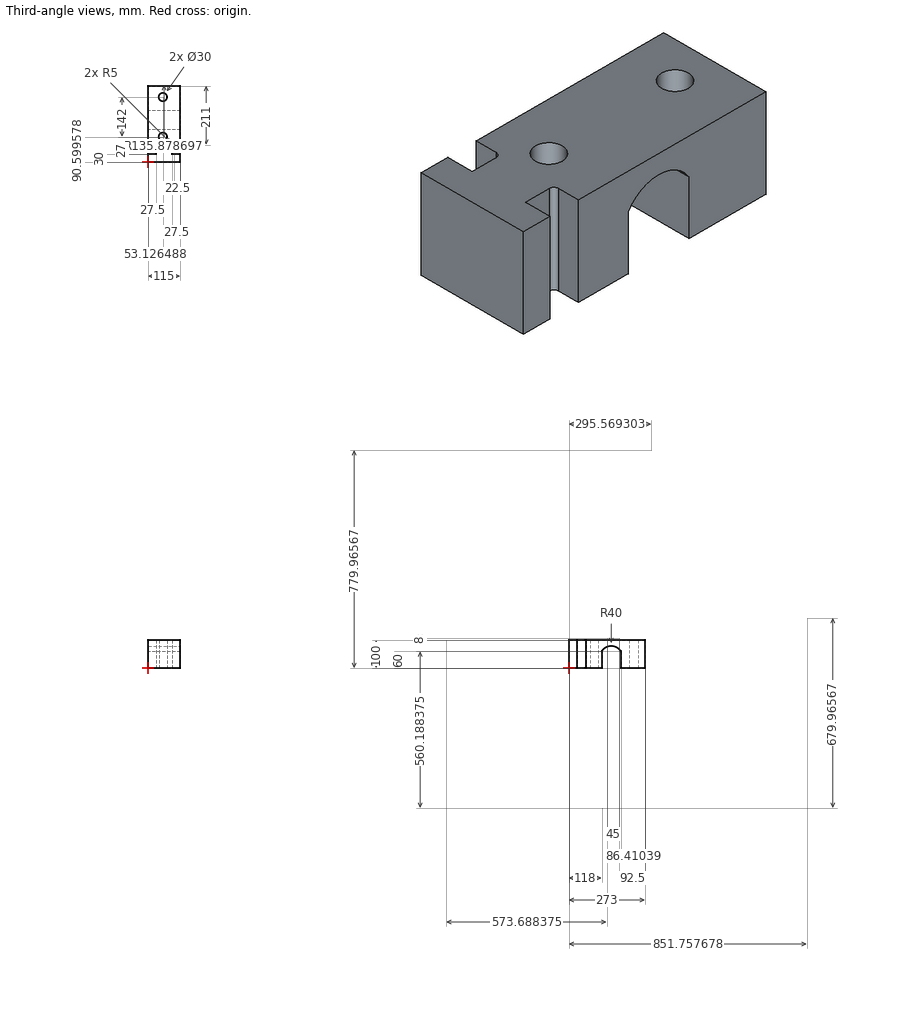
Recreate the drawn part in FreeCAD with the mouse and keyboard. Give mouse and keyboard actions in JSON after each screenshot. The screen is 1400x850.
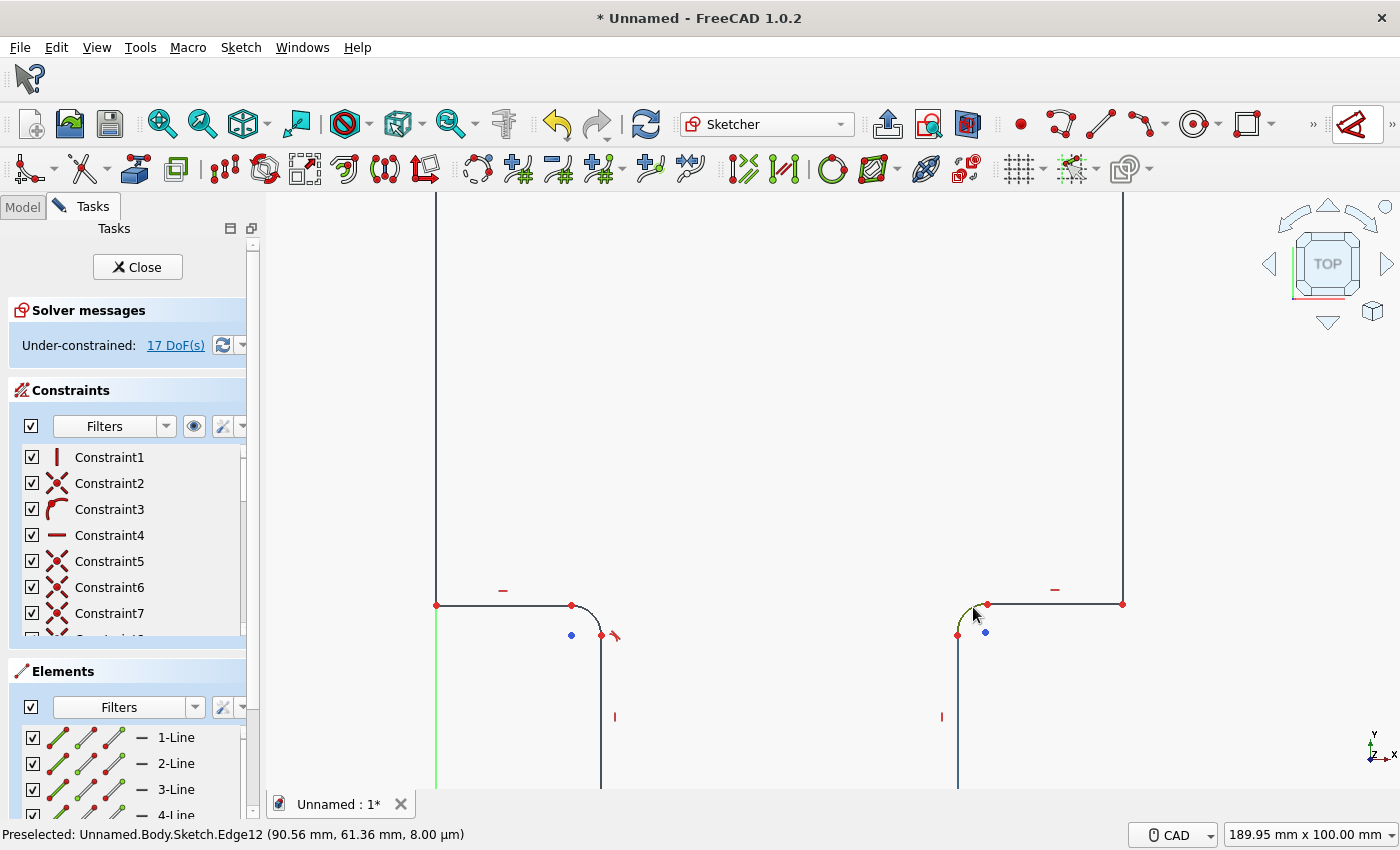
{"action": "key", "text": "t"}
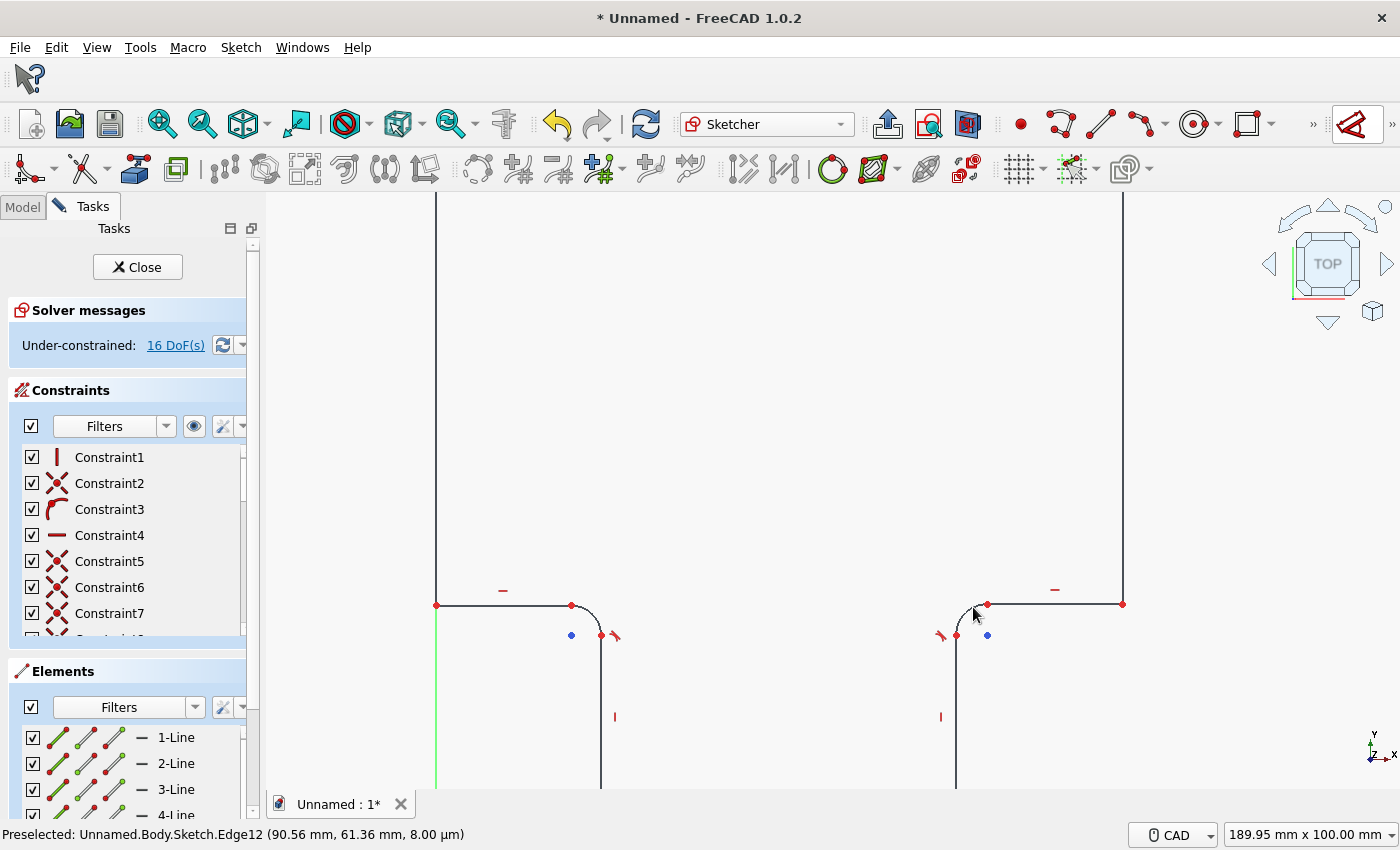
{"action": "scroll", "coordinate": [760, 612], "scroll_direction": "down", "scroll_amount": 7}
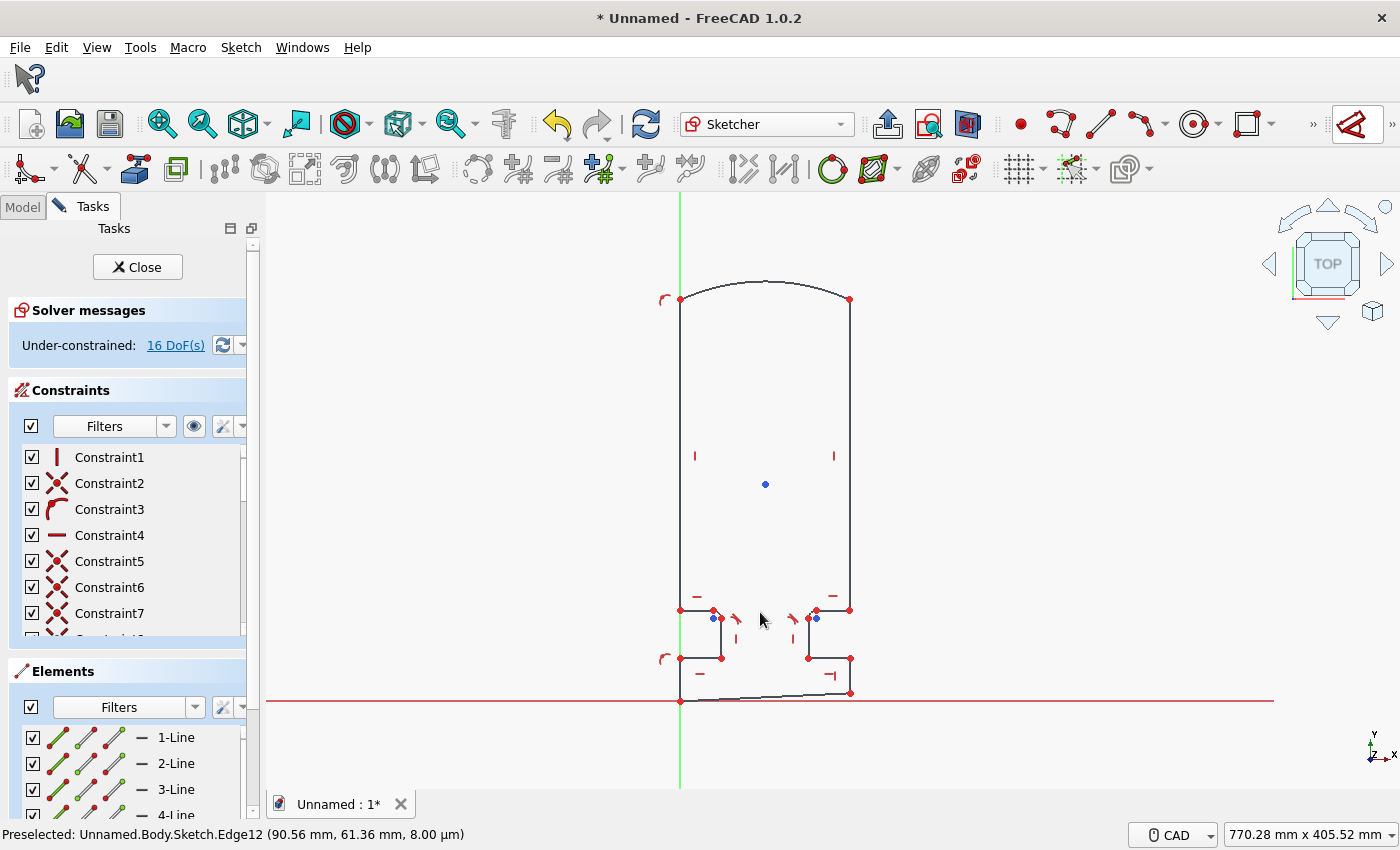
{"action": "scroll", "coordinate": [826, 611], "scroll_direction": "up", "scroll_amount": 2}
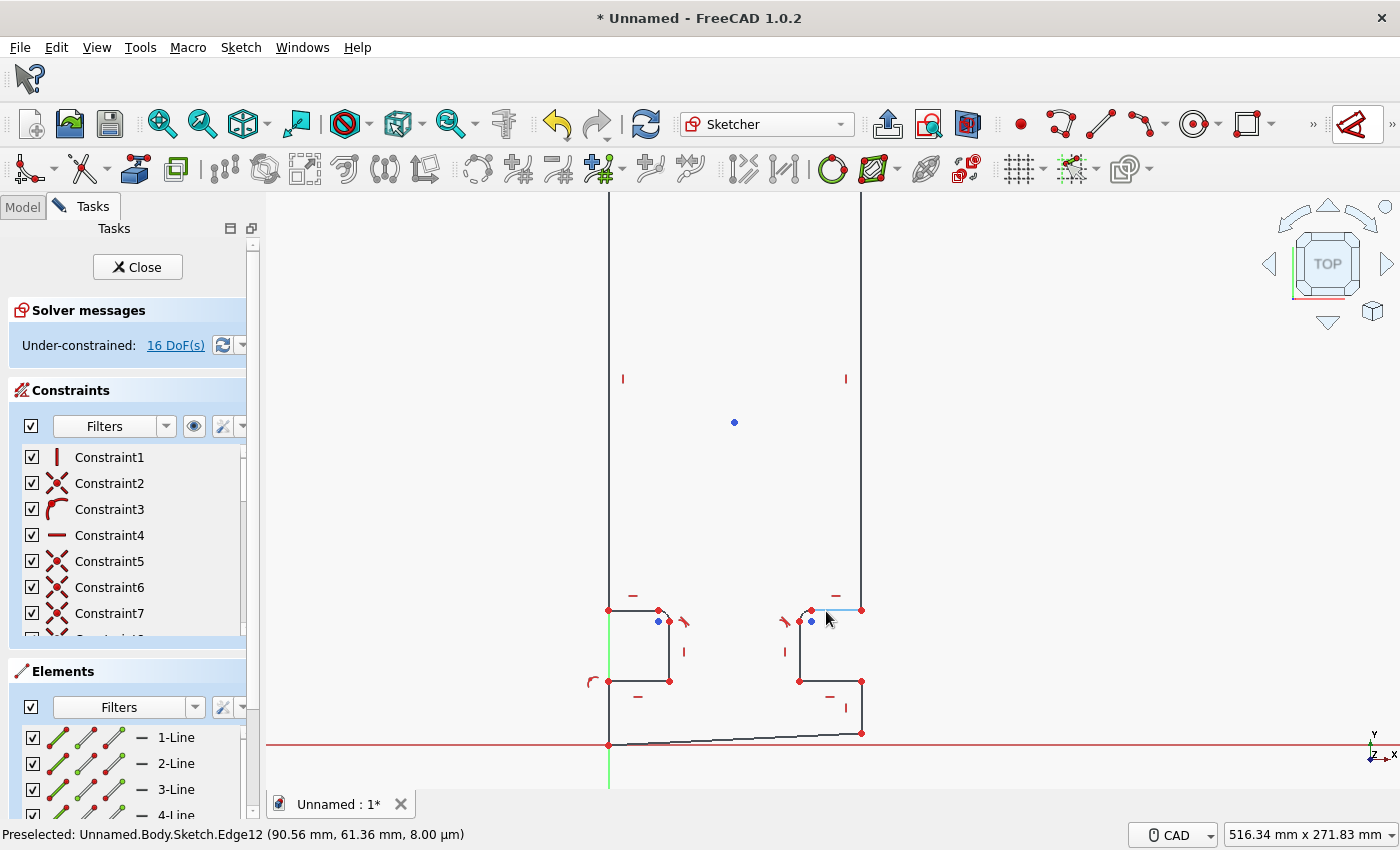
{"action": "left_click", "coordinate": [826, 610]}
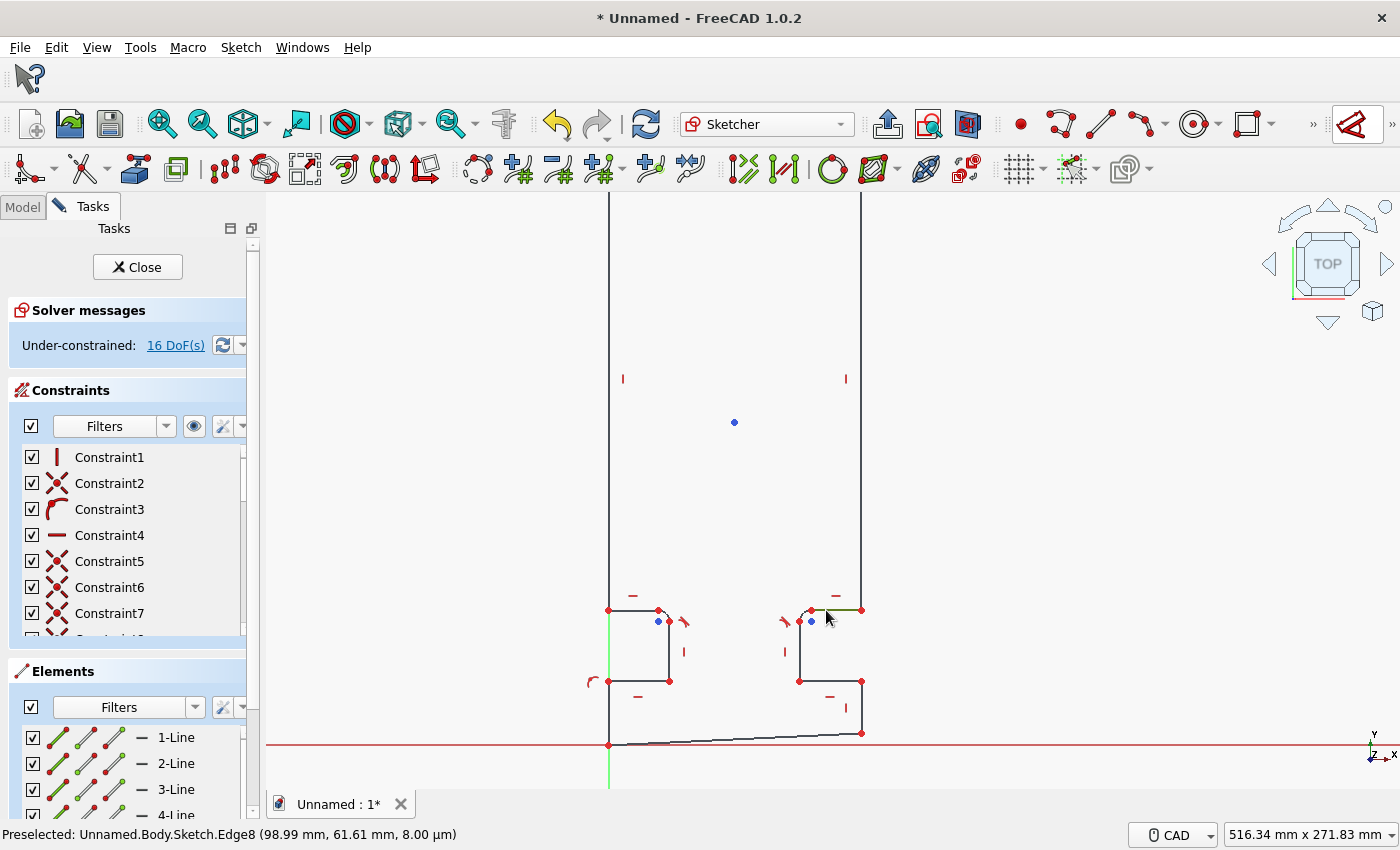
{"action": "scroll", "coordinate": [803, 613], "scroll_direction": "up", "scroll_amount": 3}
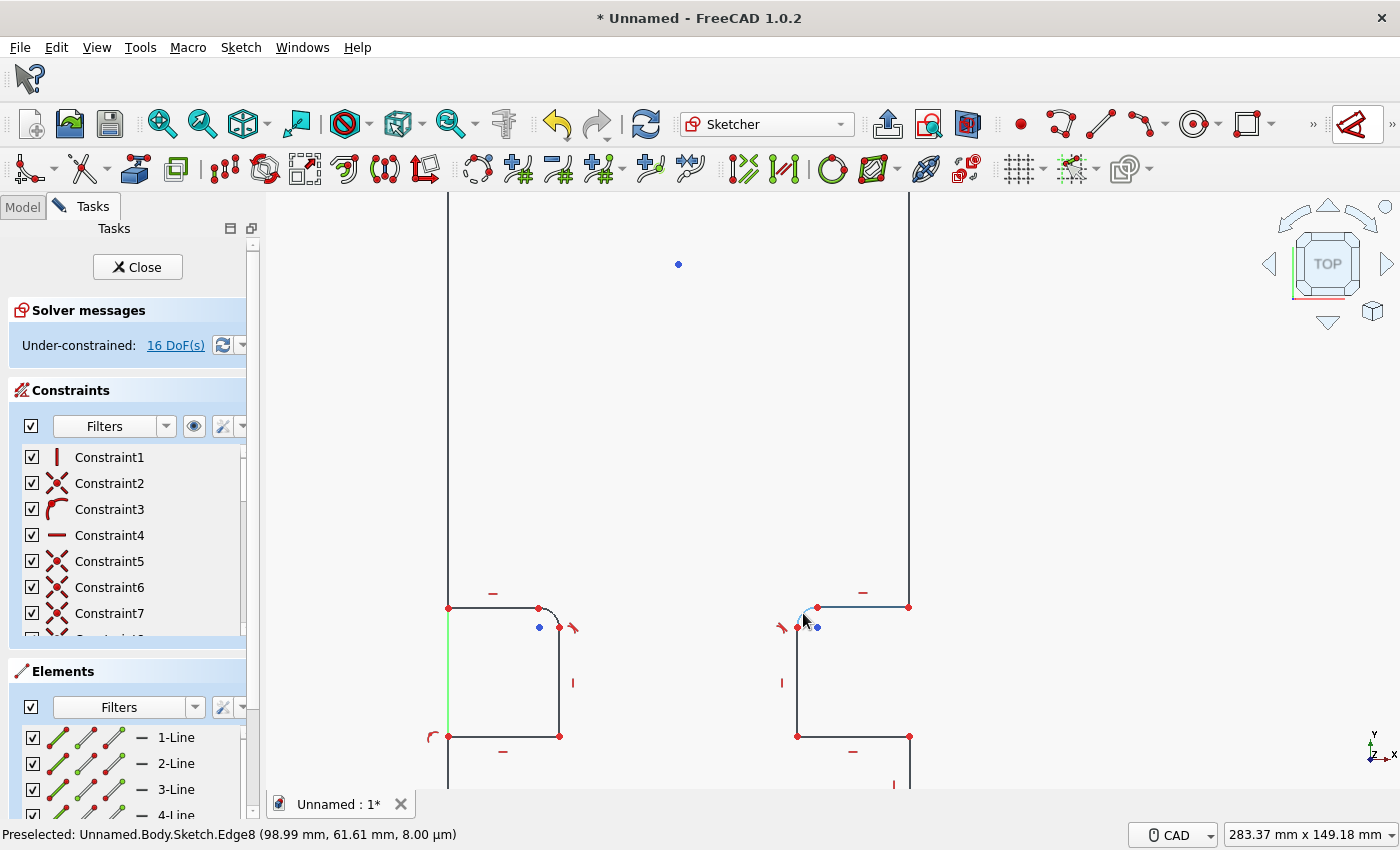
{"action": "left_click", "coordinate": [803, 613]}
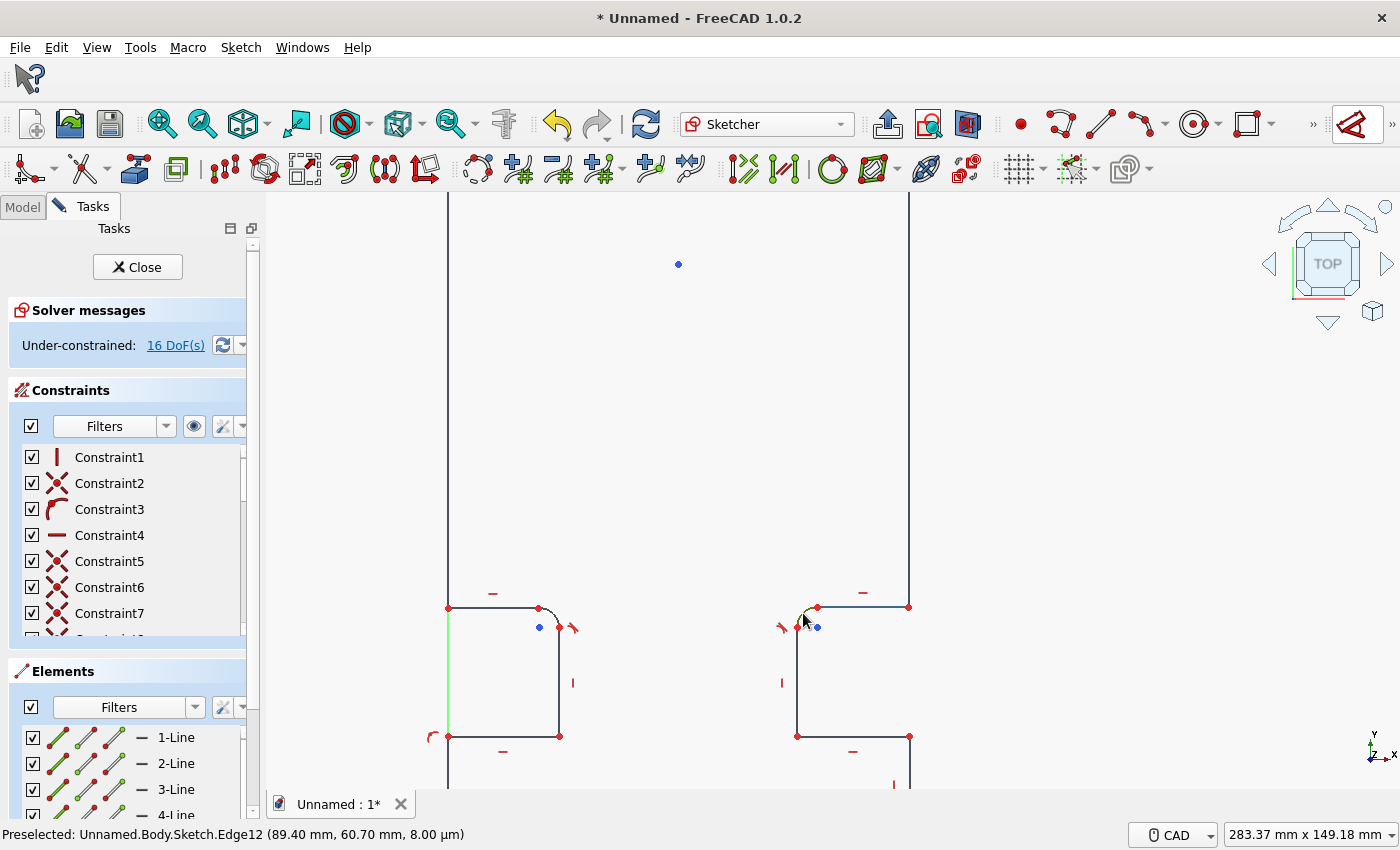
{"action": "key", "text": "t"}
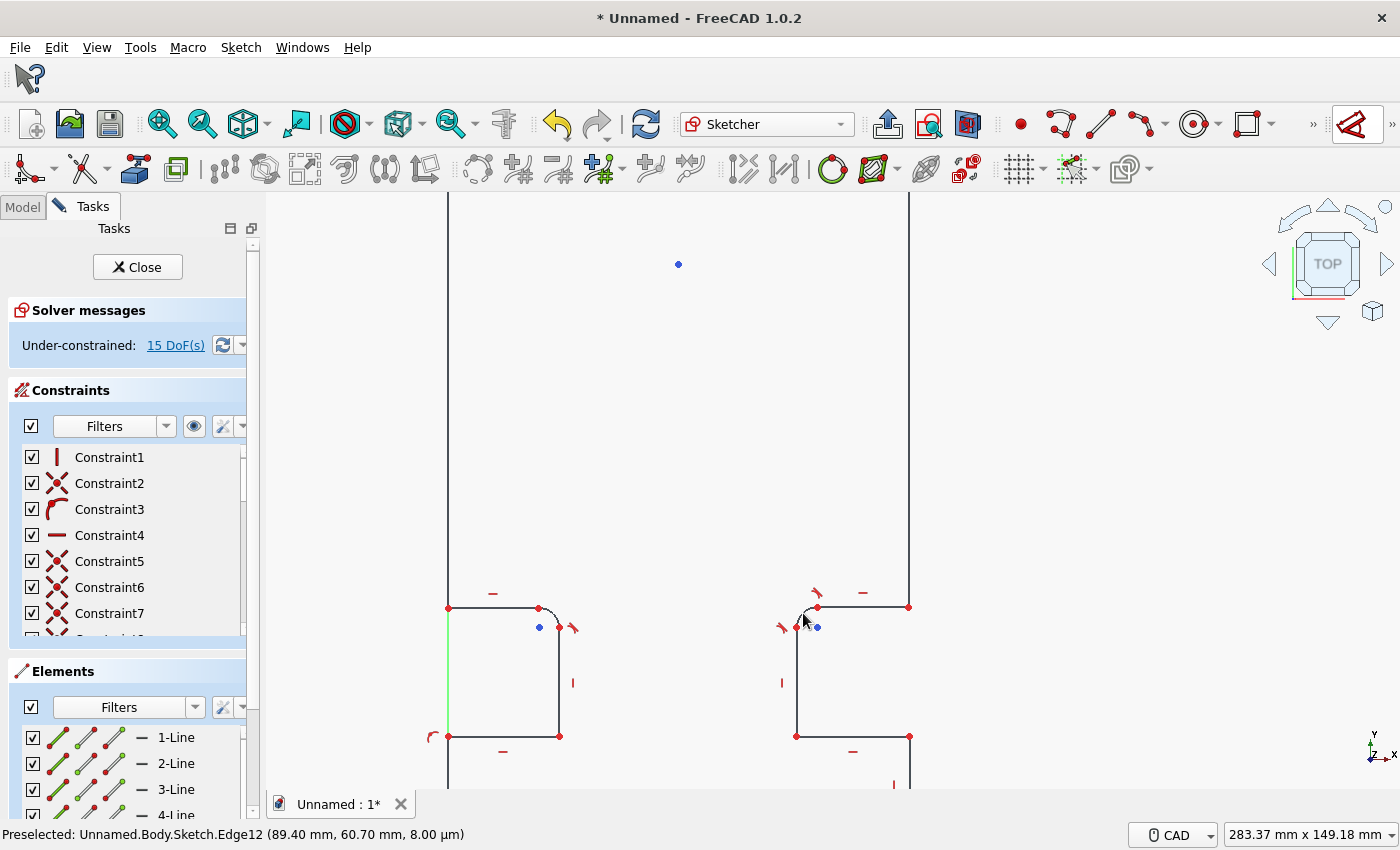
{"action": "left_click", "coordinate": [476, 608]}